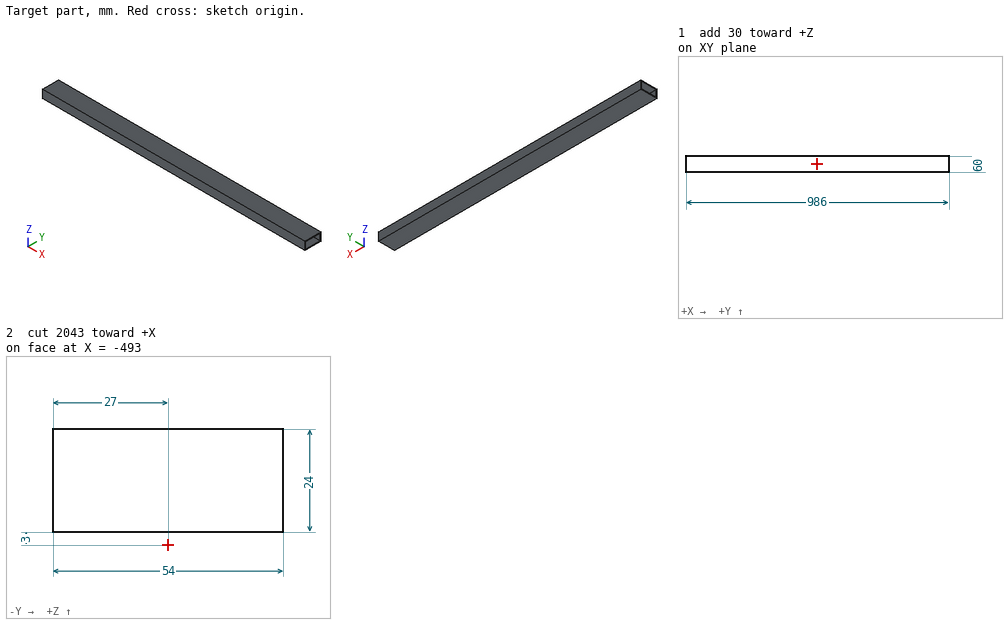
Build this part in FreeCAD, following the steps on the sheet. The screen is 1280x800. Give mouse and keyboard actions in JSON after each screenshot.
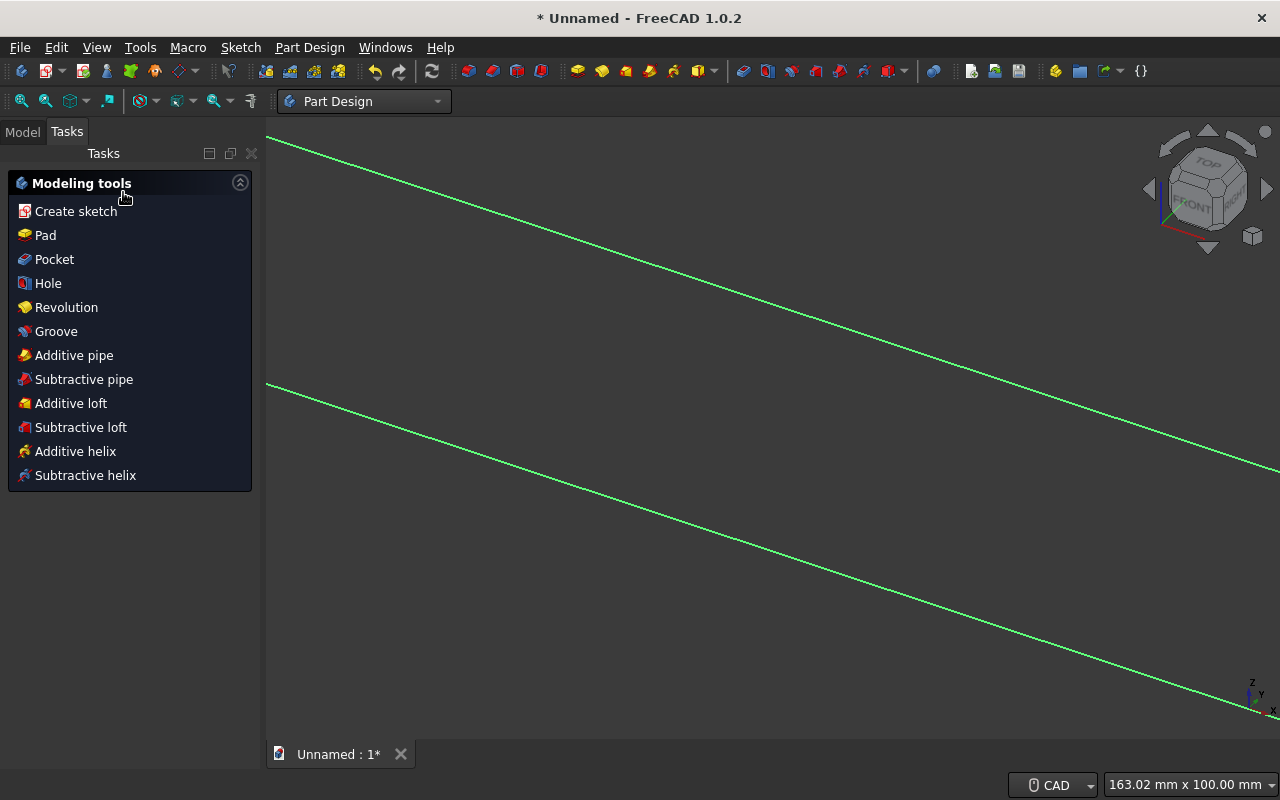
{"action": "left_click", "coordinate": [578, 72]}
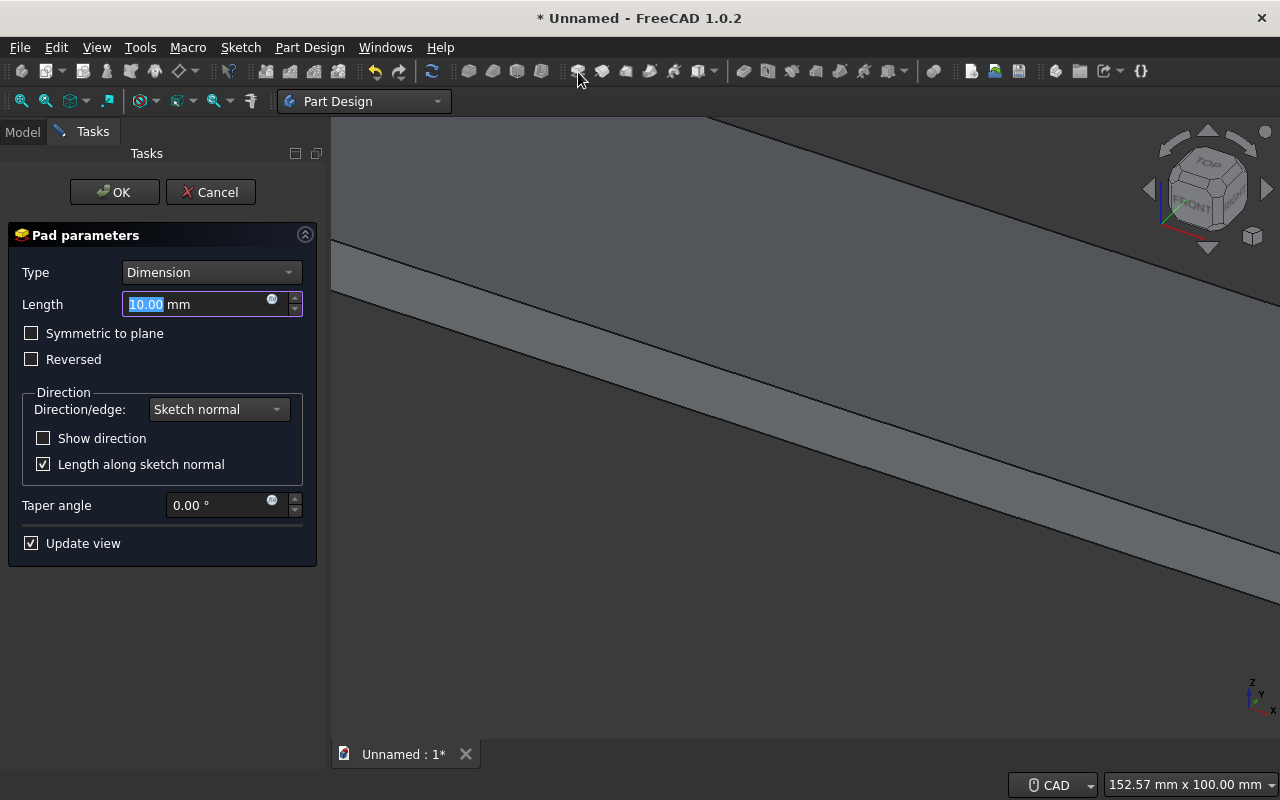
{"action": "type", "text": "30"}
{"action": "key", "text": "Tab"}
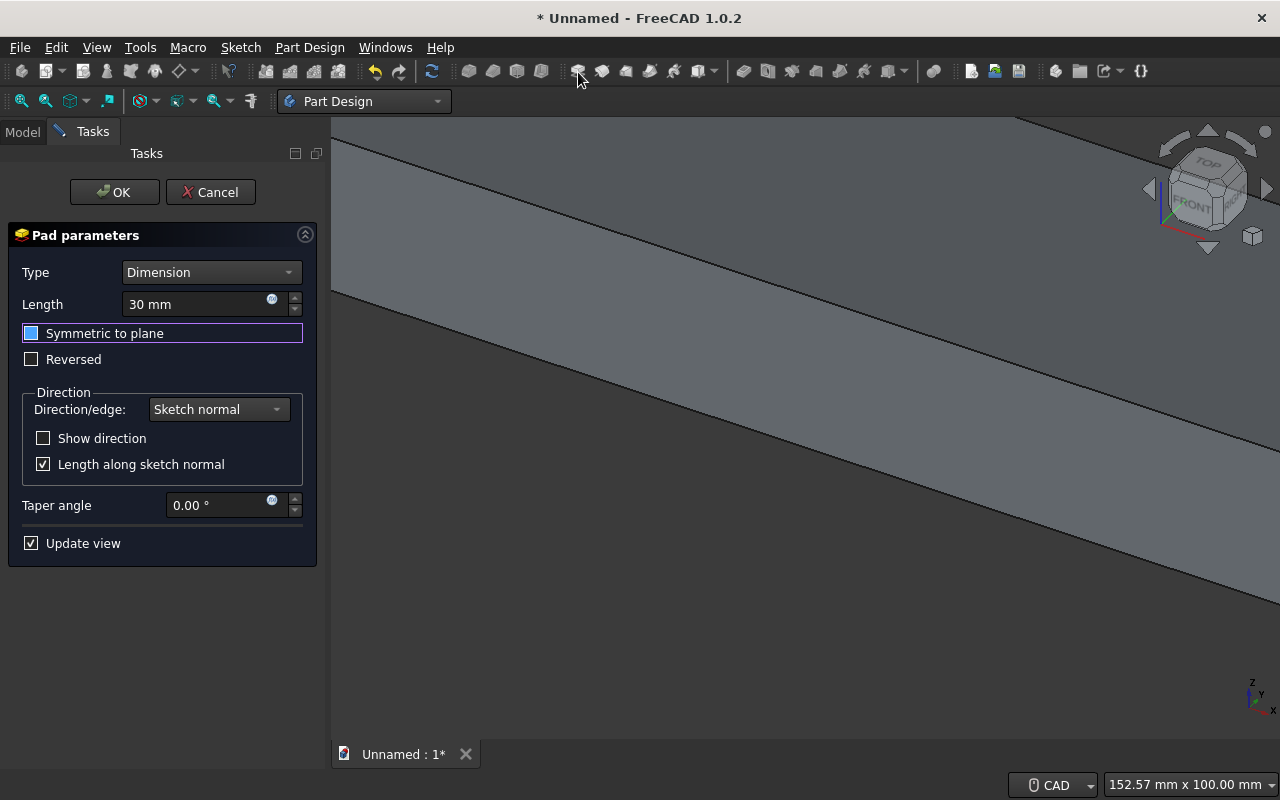
{"action": "left_click", "coordinate": [115, 192]}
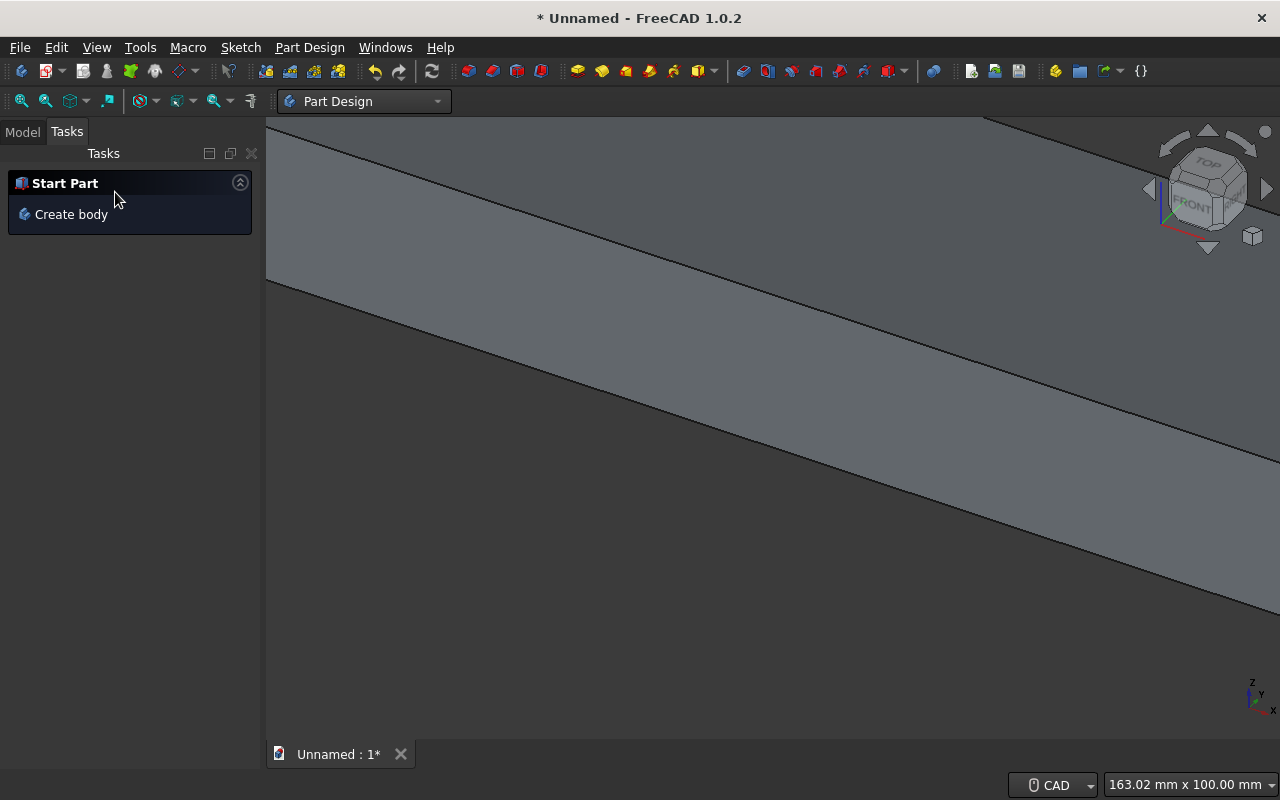
{"action": "left_click", "coordinate": [22, 102]}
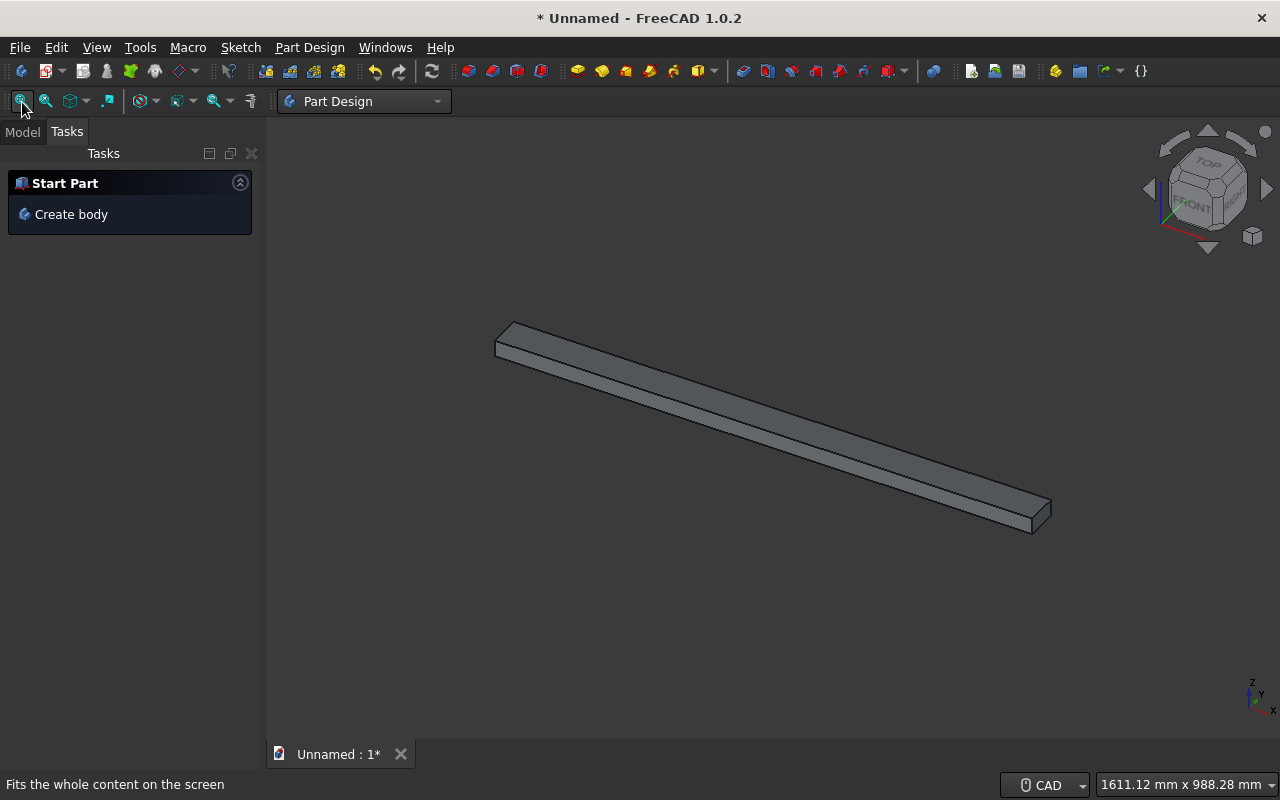
{"action": "key", "text": "6"}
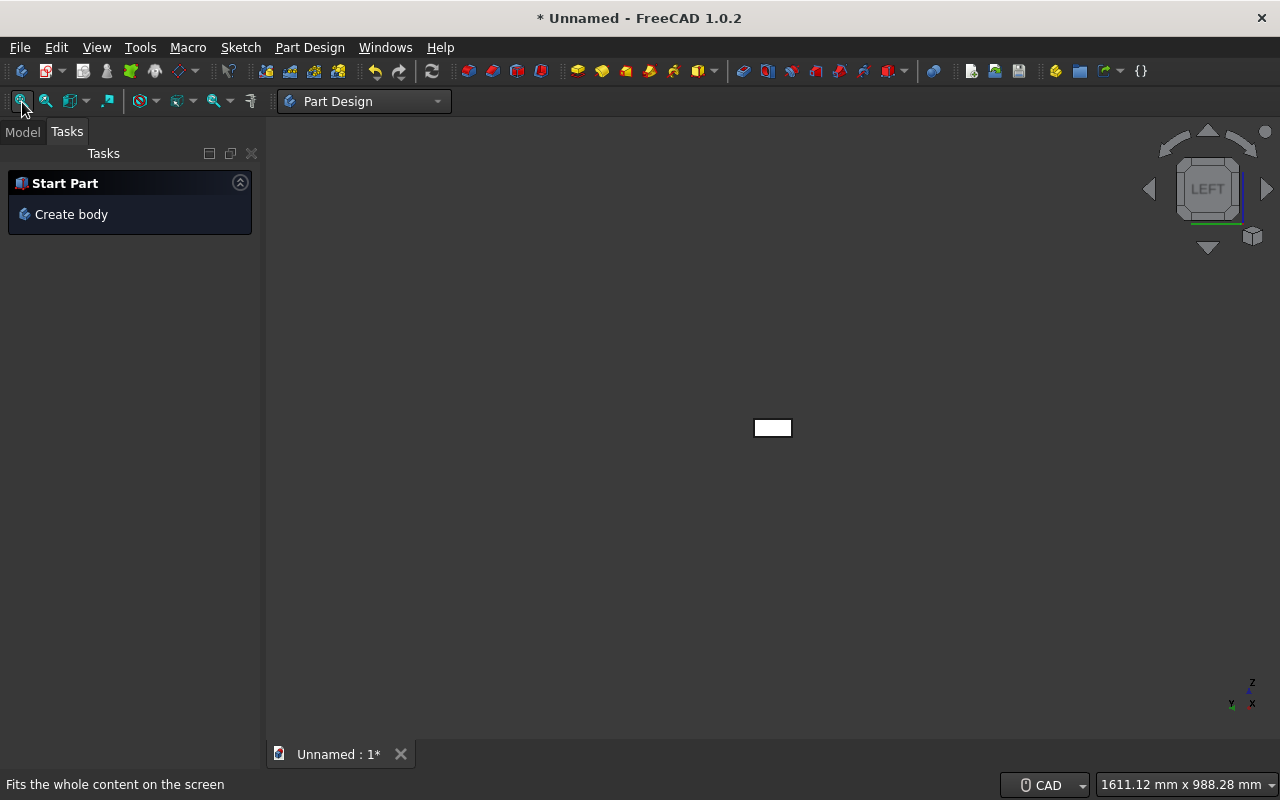
{"action": "left_click", "coordinate": [22, 102]}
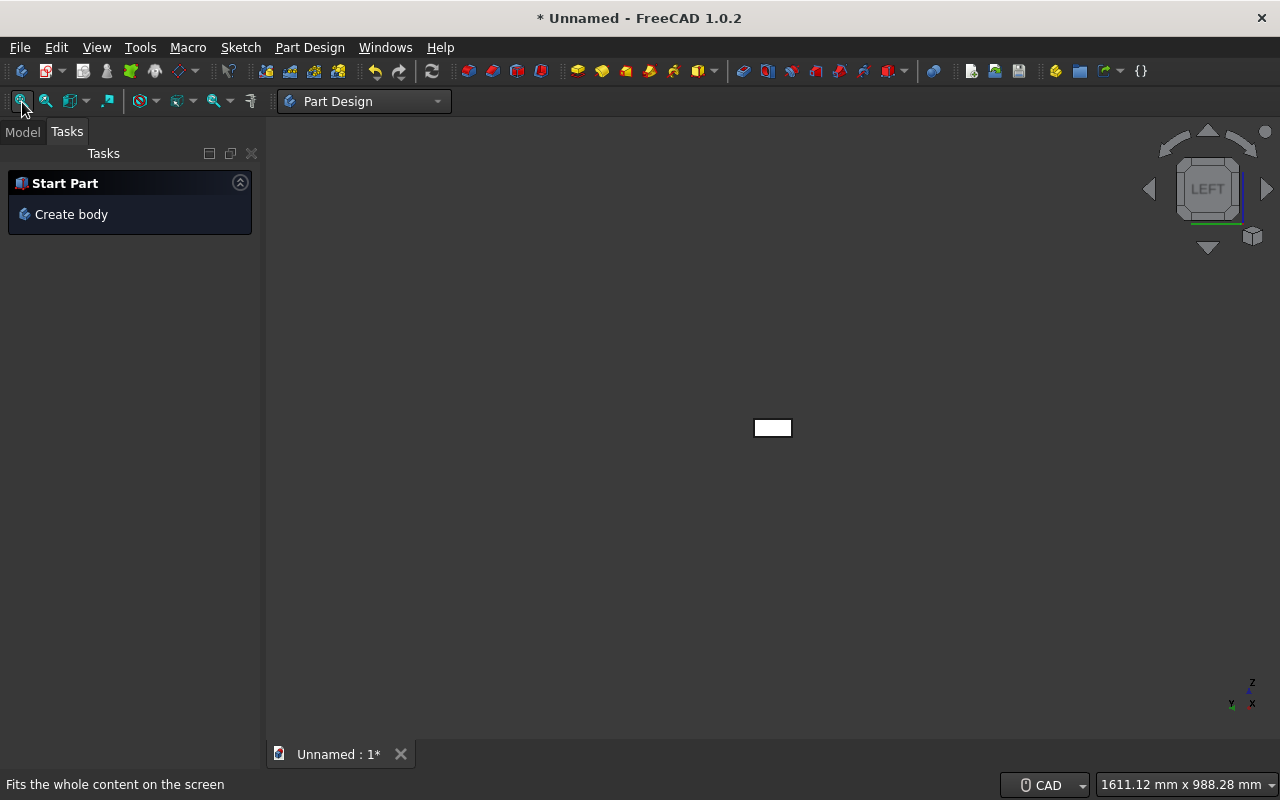
{"action": "left_click", "coordinate": [768, 427]}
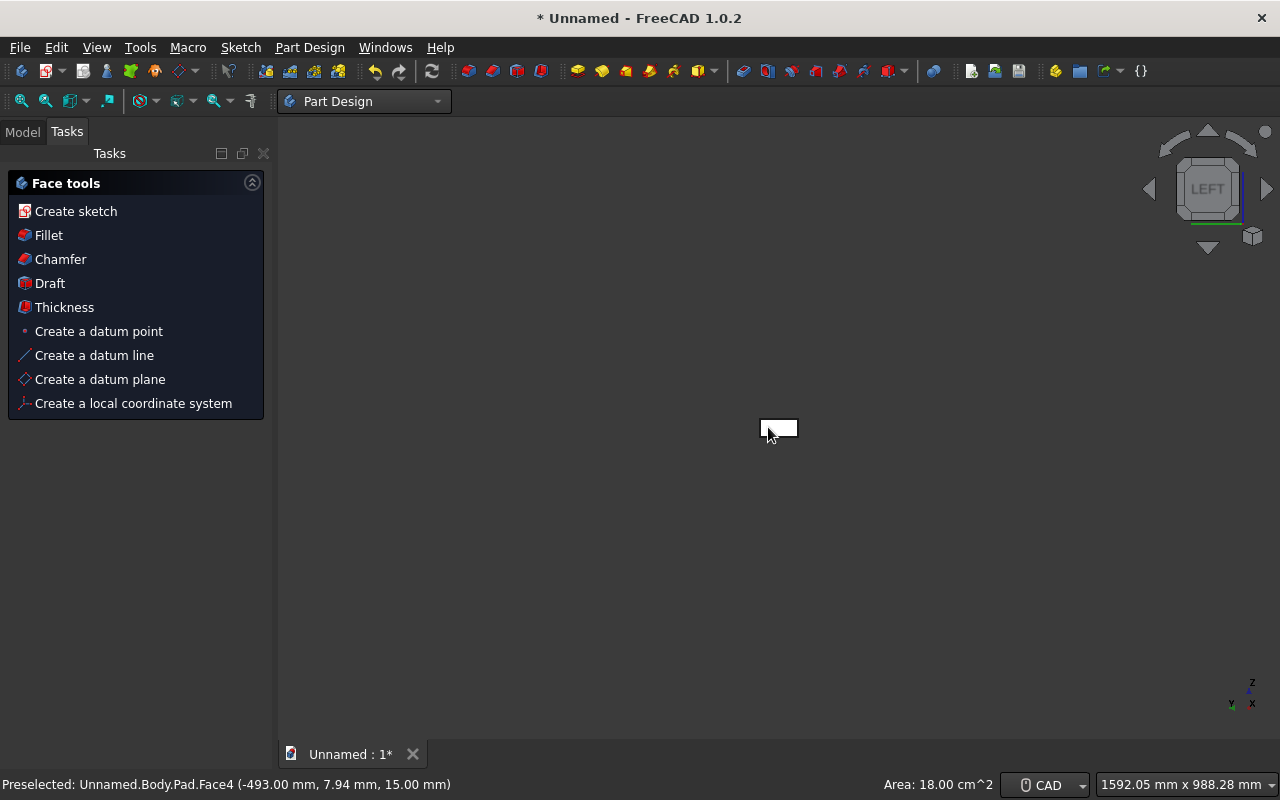
{"action": "left_click", "coordinate": [46, 72]}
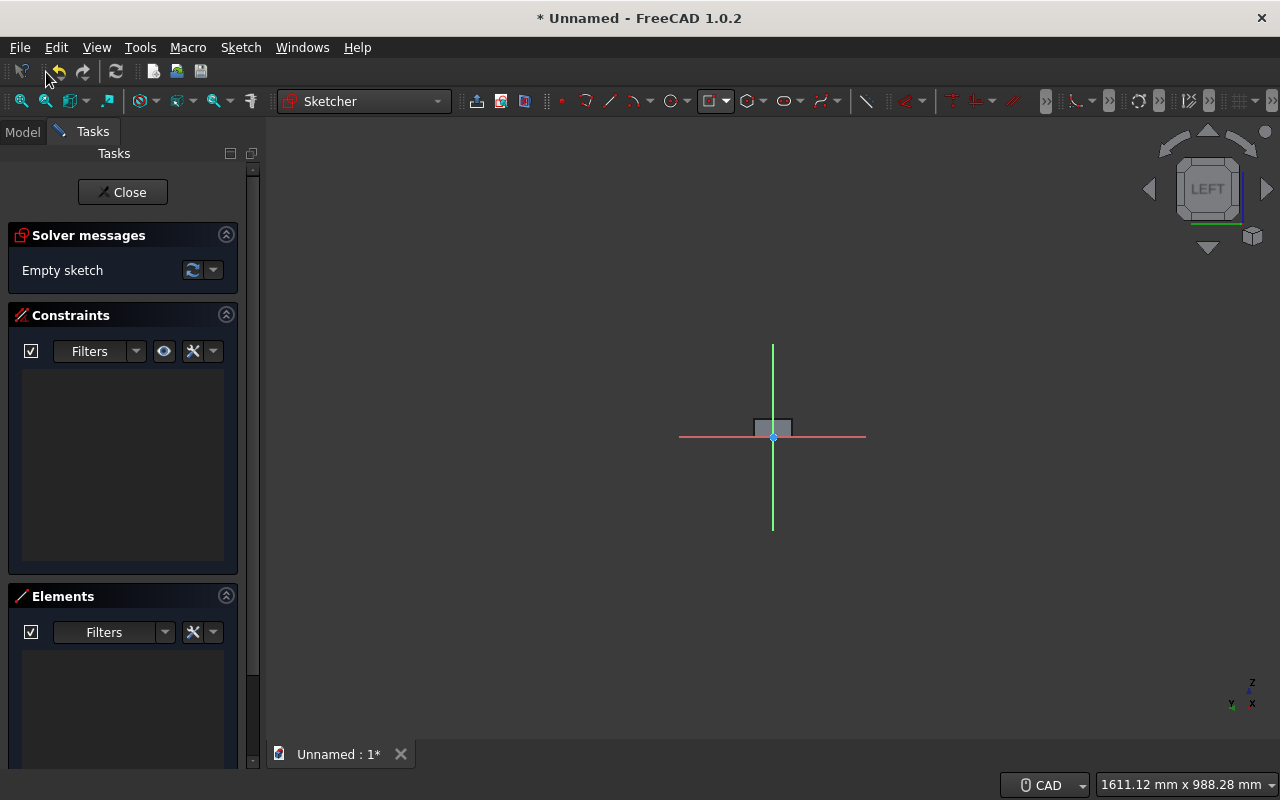
{"action": "scroll", "coordinate": [777, 429], "scroll_direction": "up", "scroll_amount": 14}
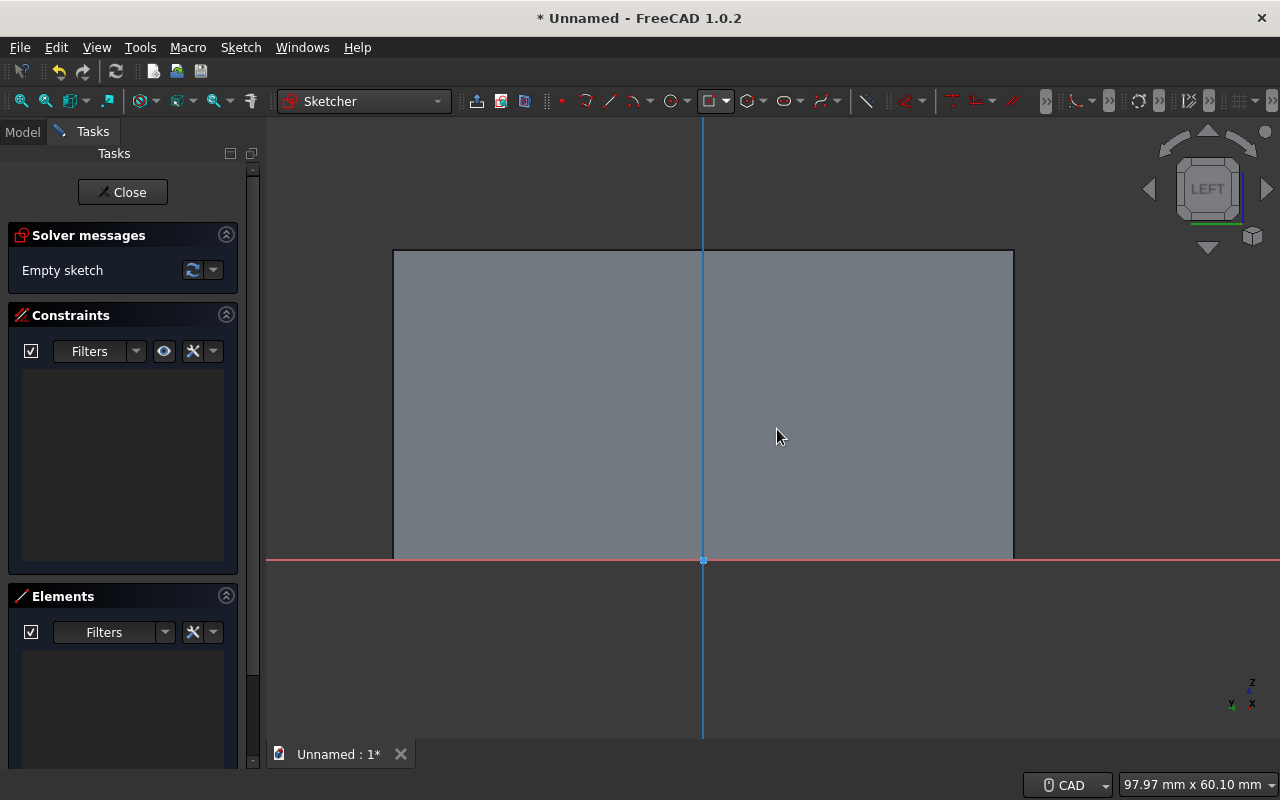
{"action": "key", "text": "g r"}